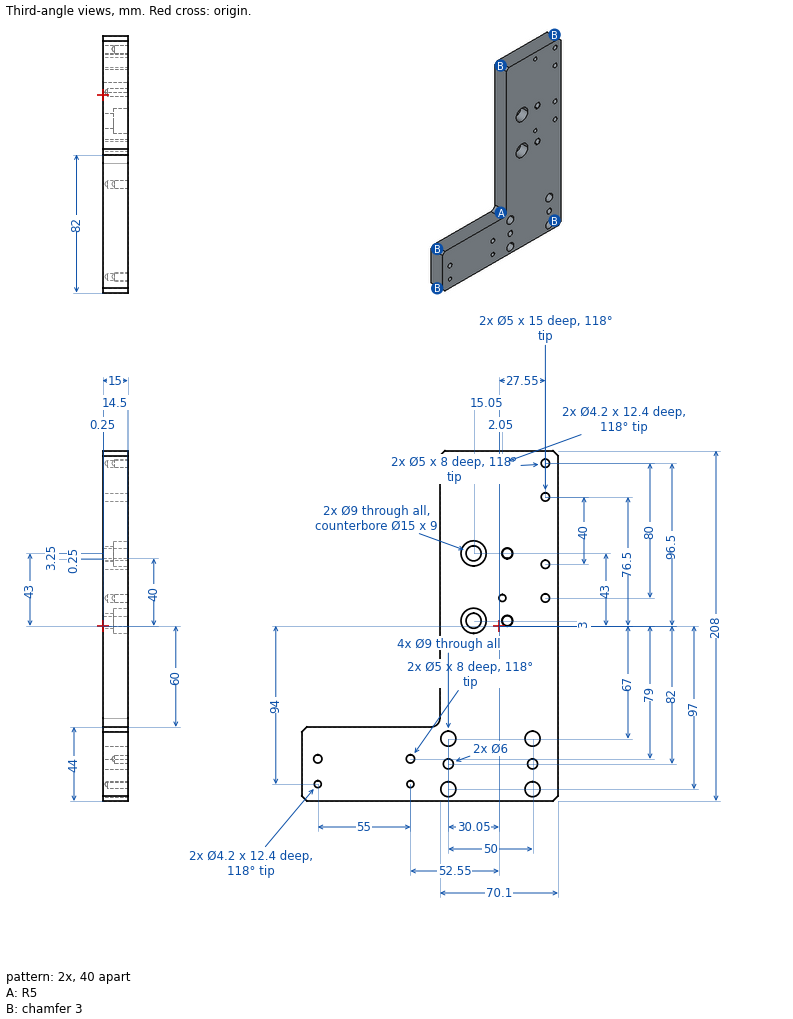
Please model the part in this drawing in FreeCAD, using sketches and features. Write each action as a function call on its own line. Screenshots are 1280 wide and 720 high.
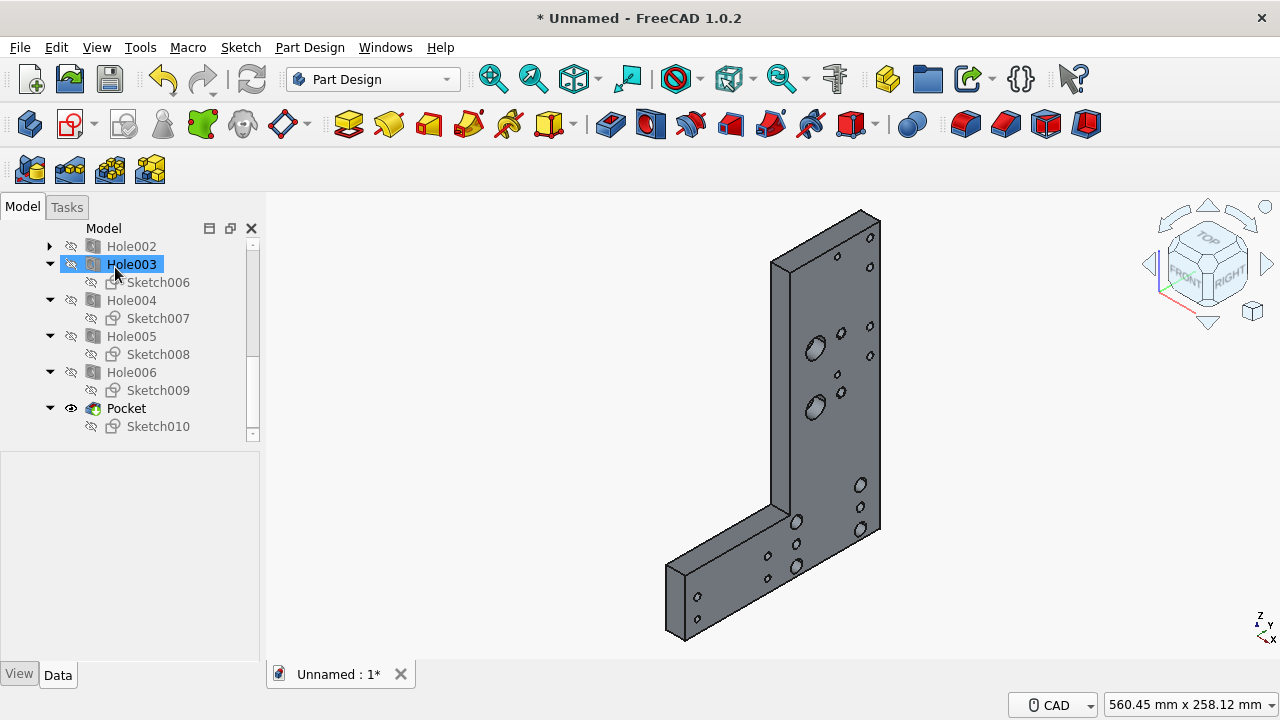
key(2)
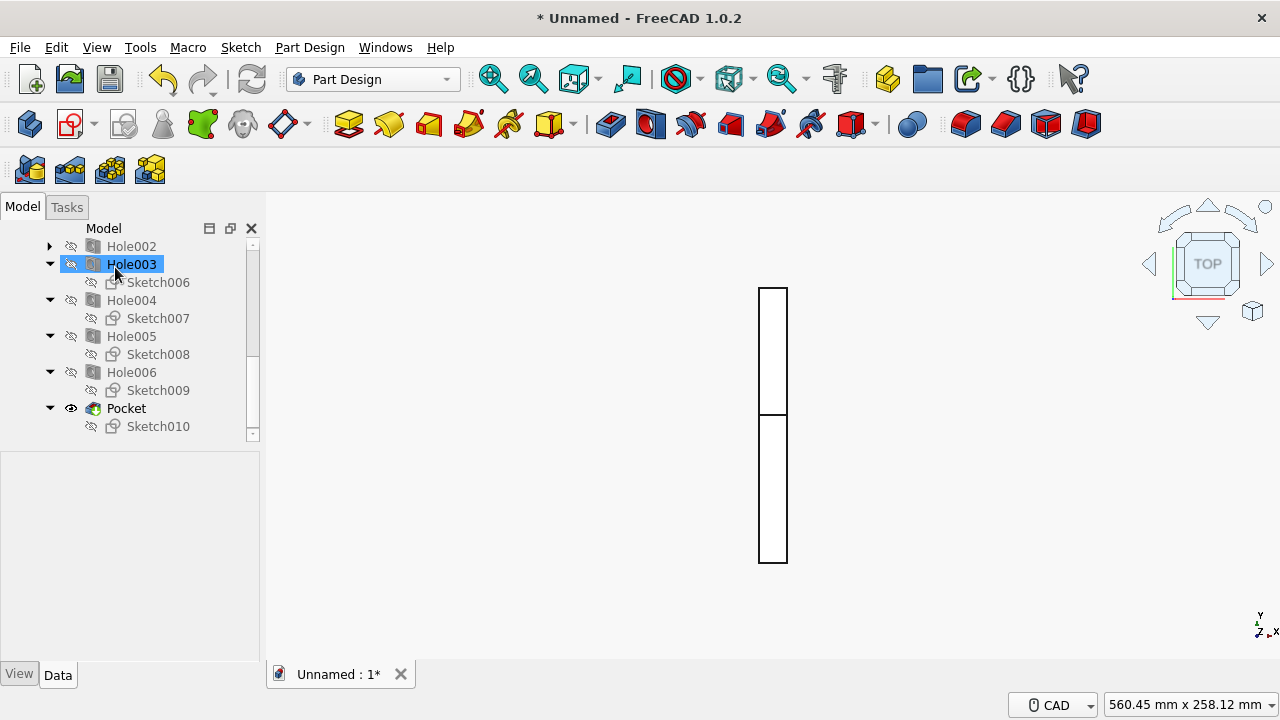
key(1)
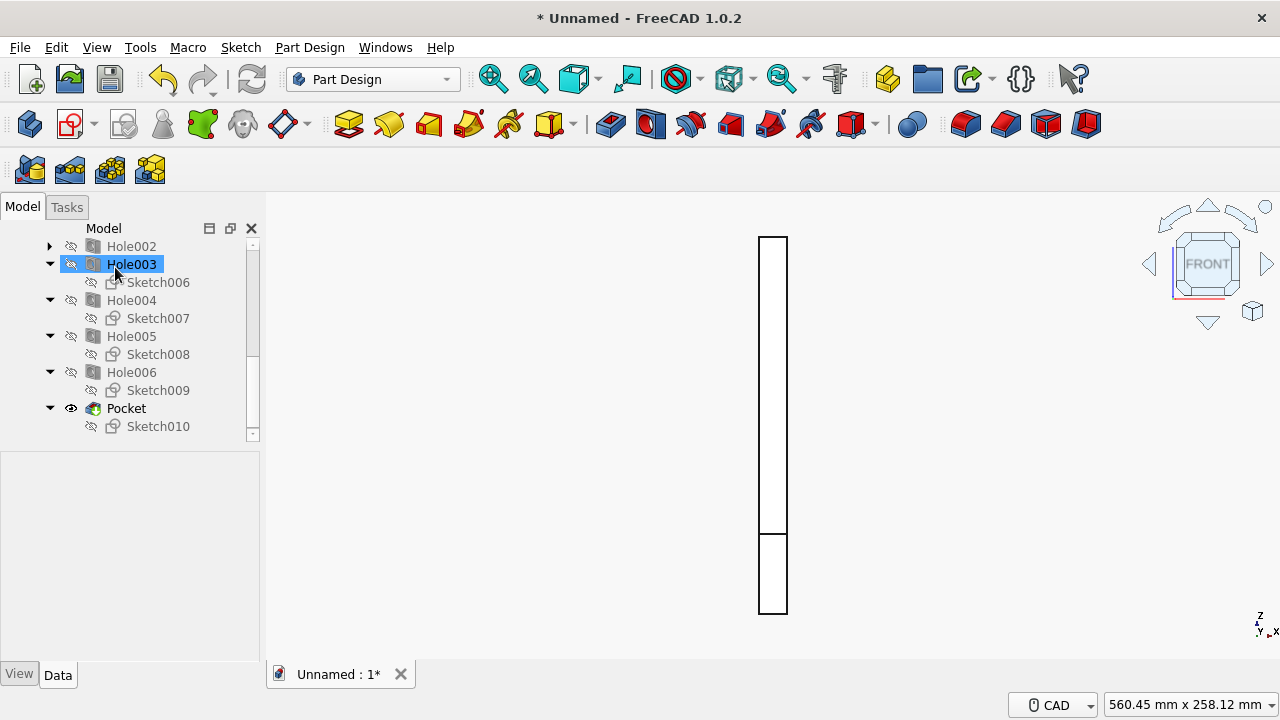
key(3)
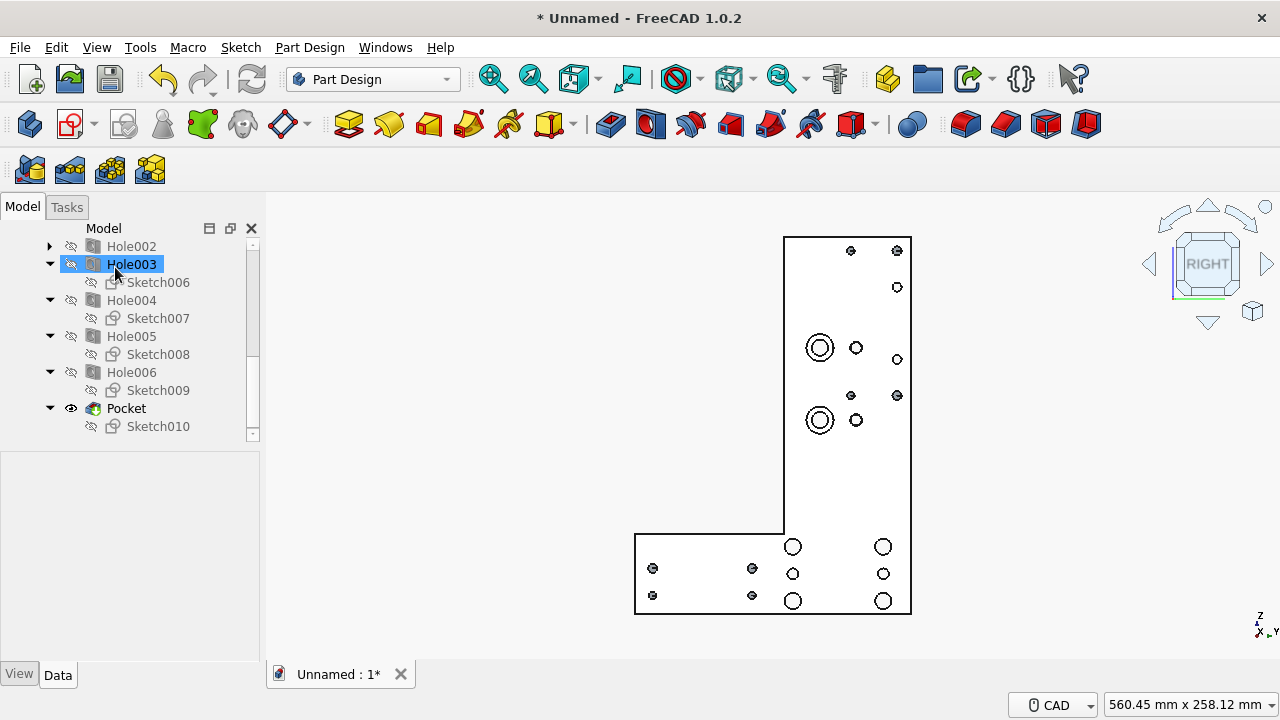
key(5)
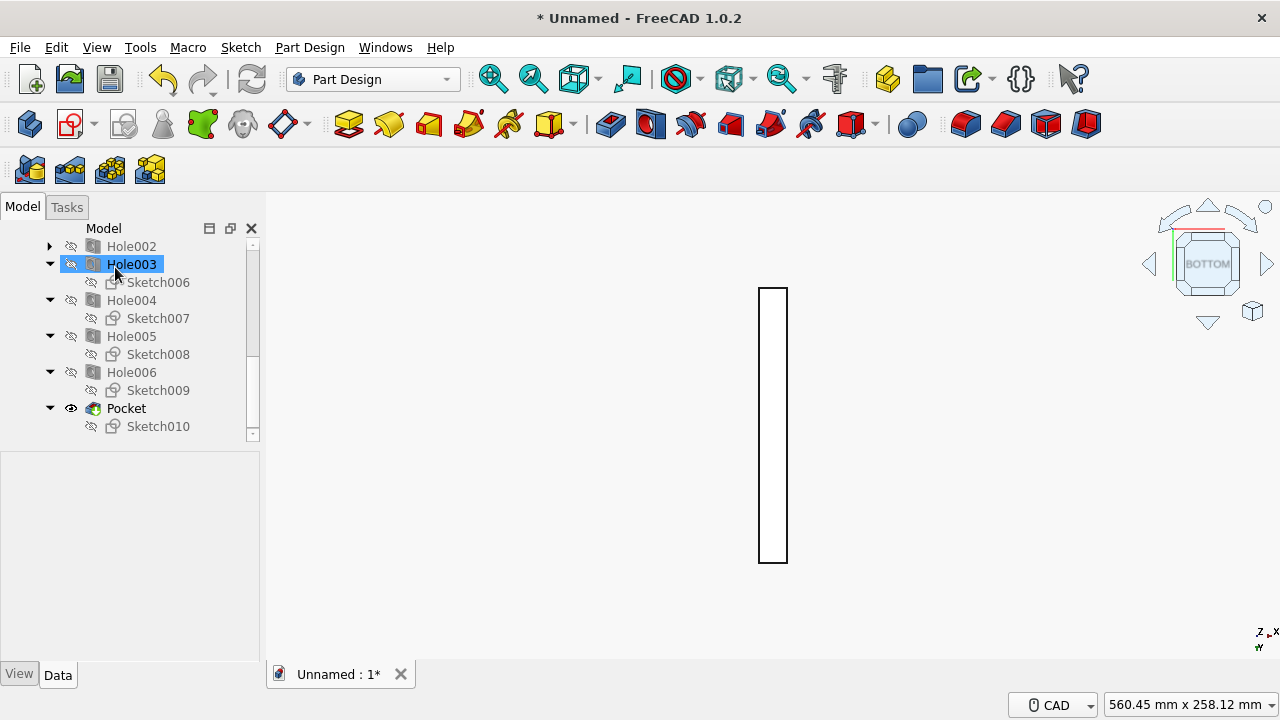
key(4)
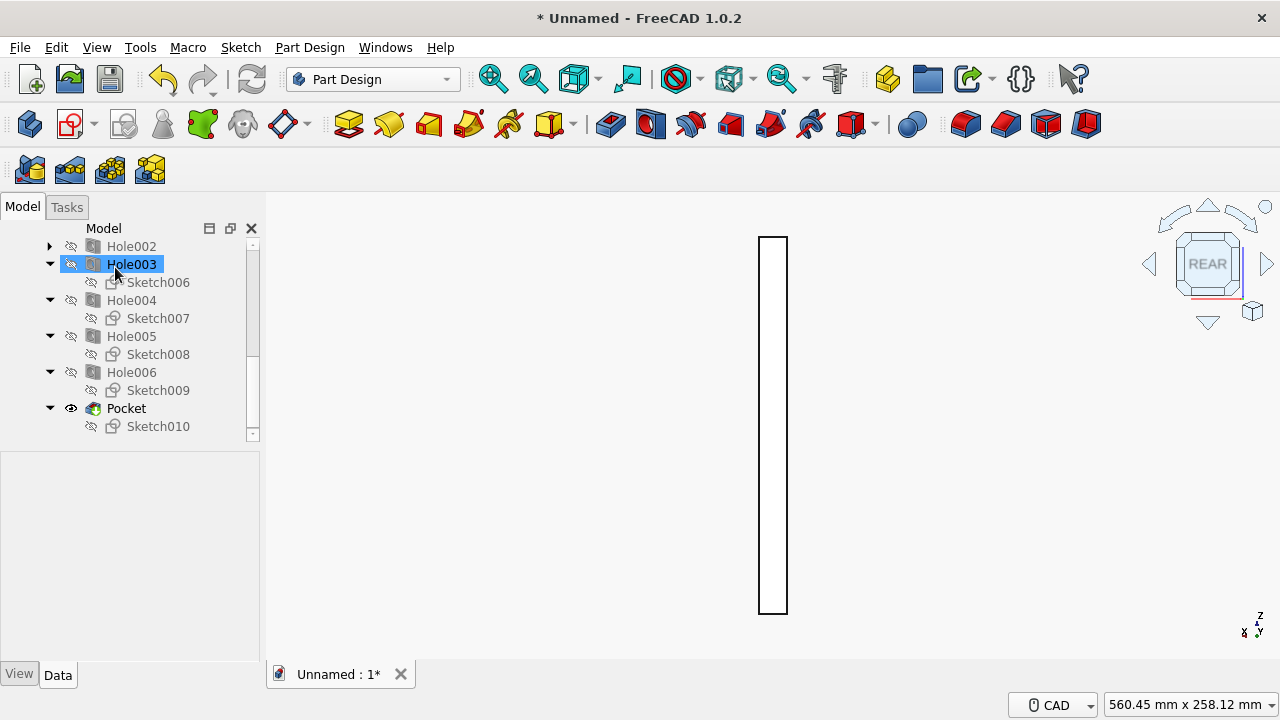
key(6)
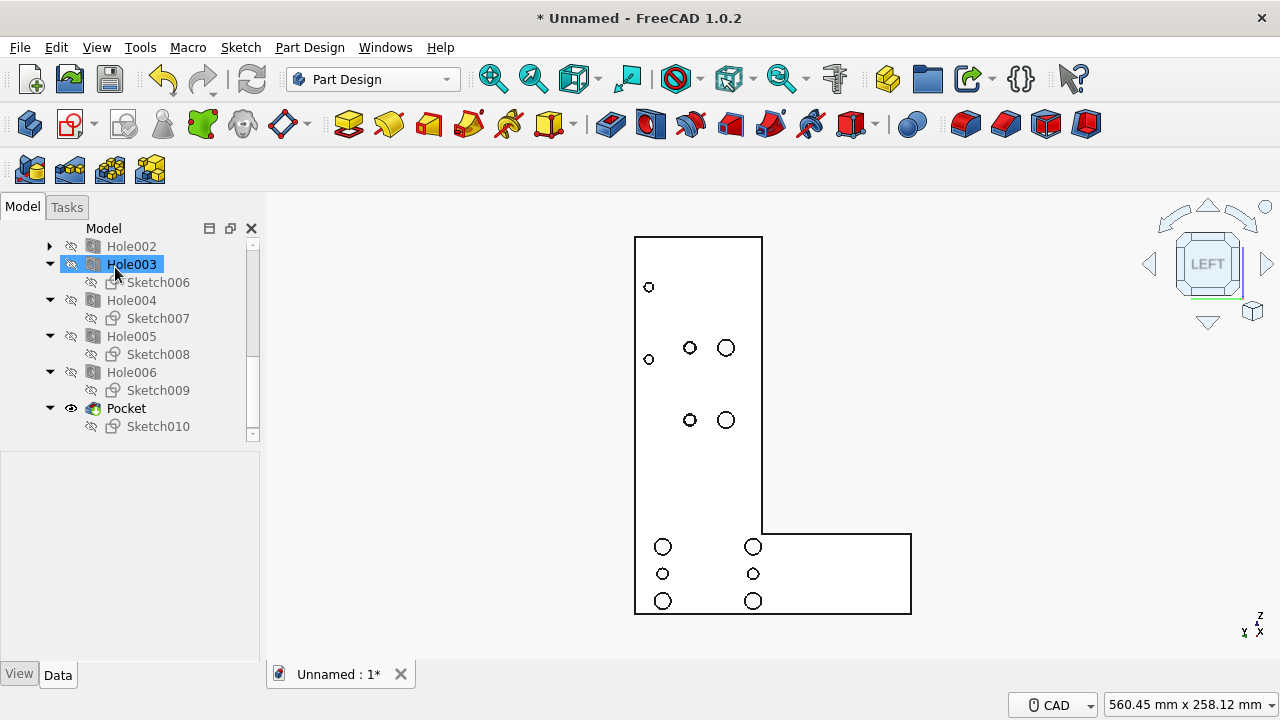
key(v)
key(3)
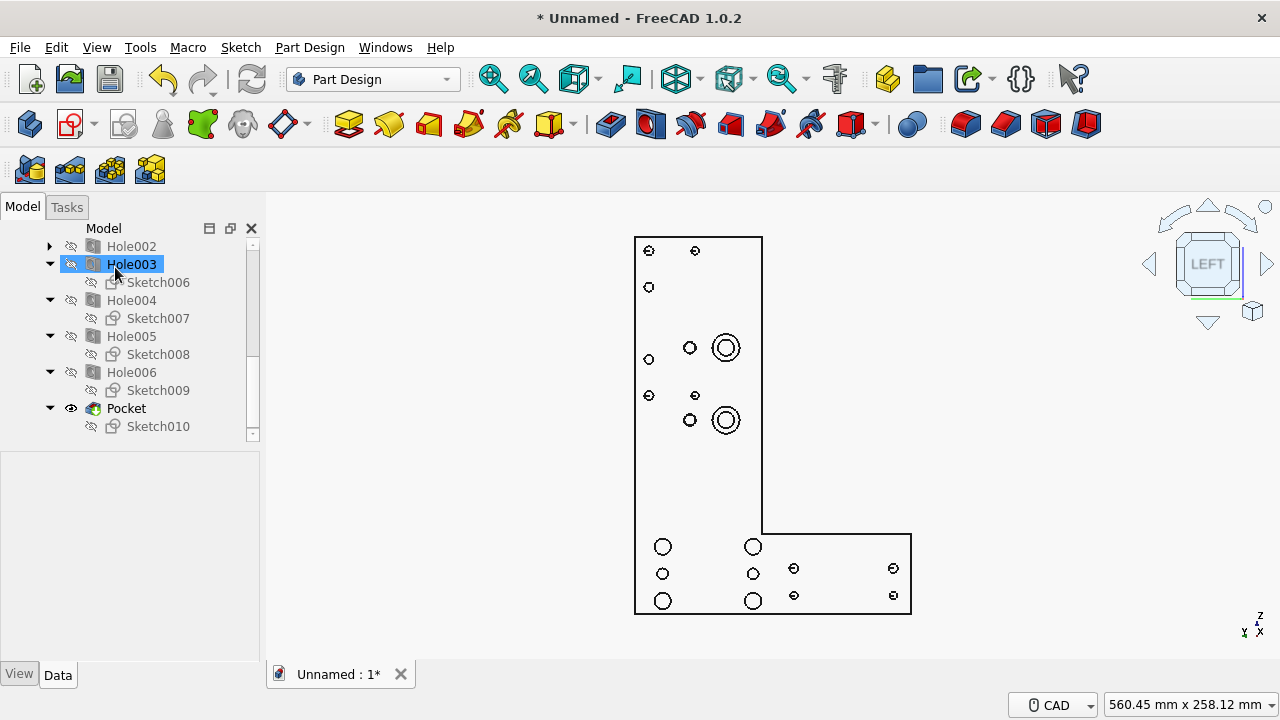
key(0)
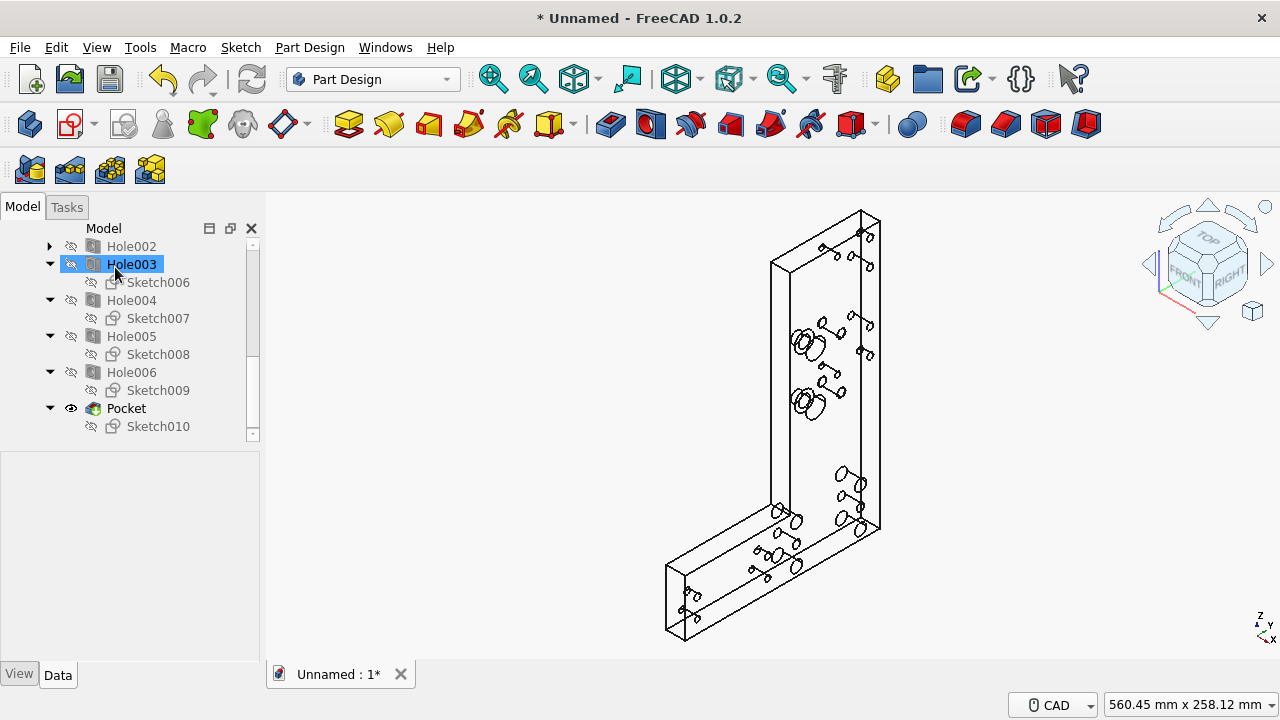
click(781, 509)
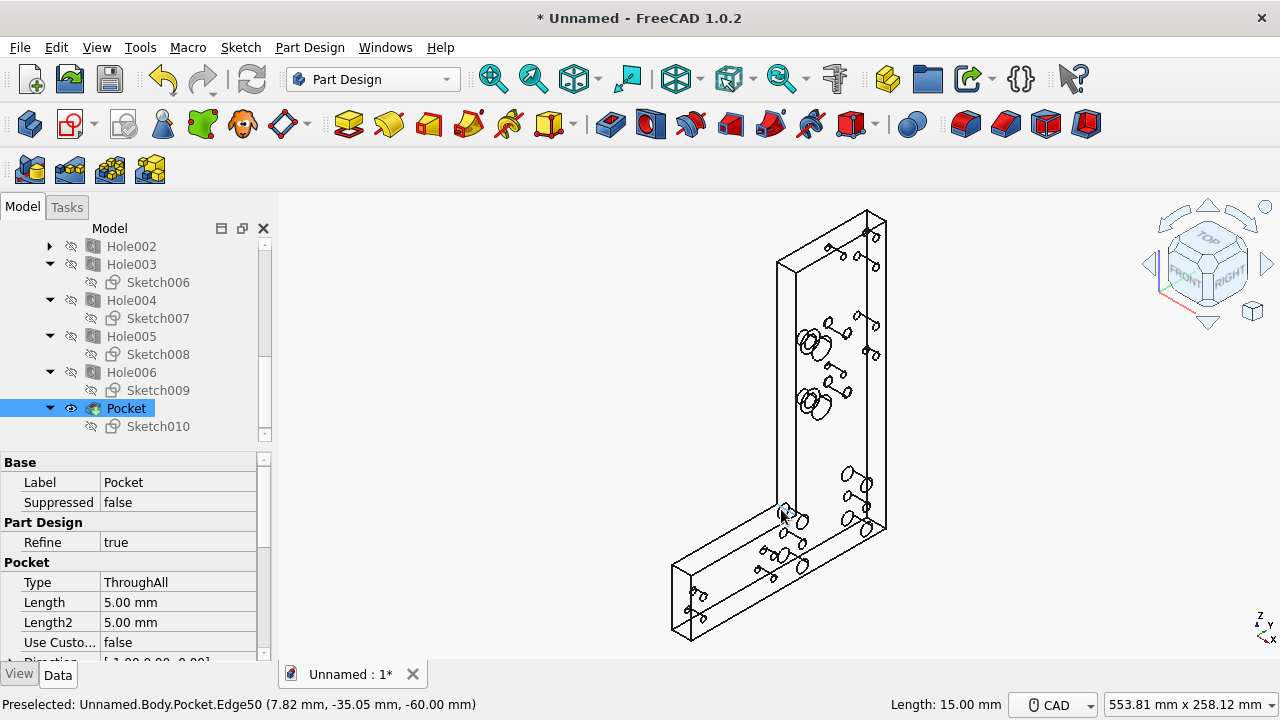
key(v)
key(1)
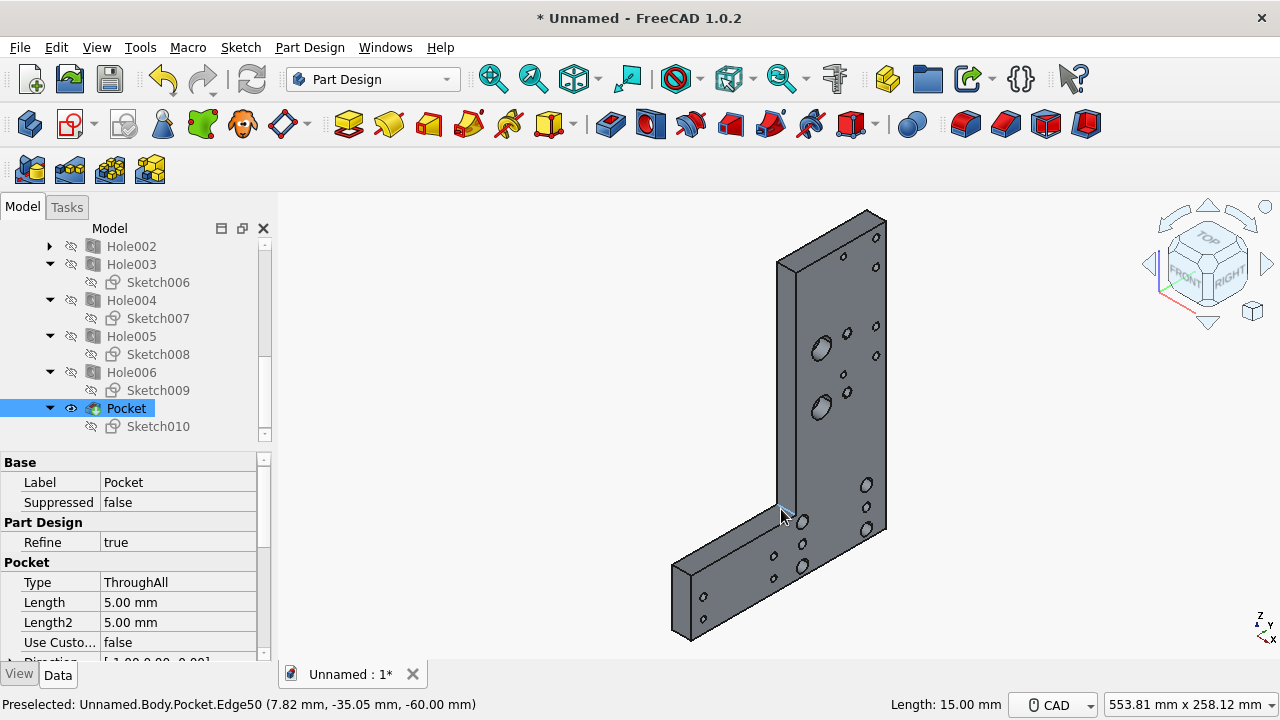
click(966, 124)